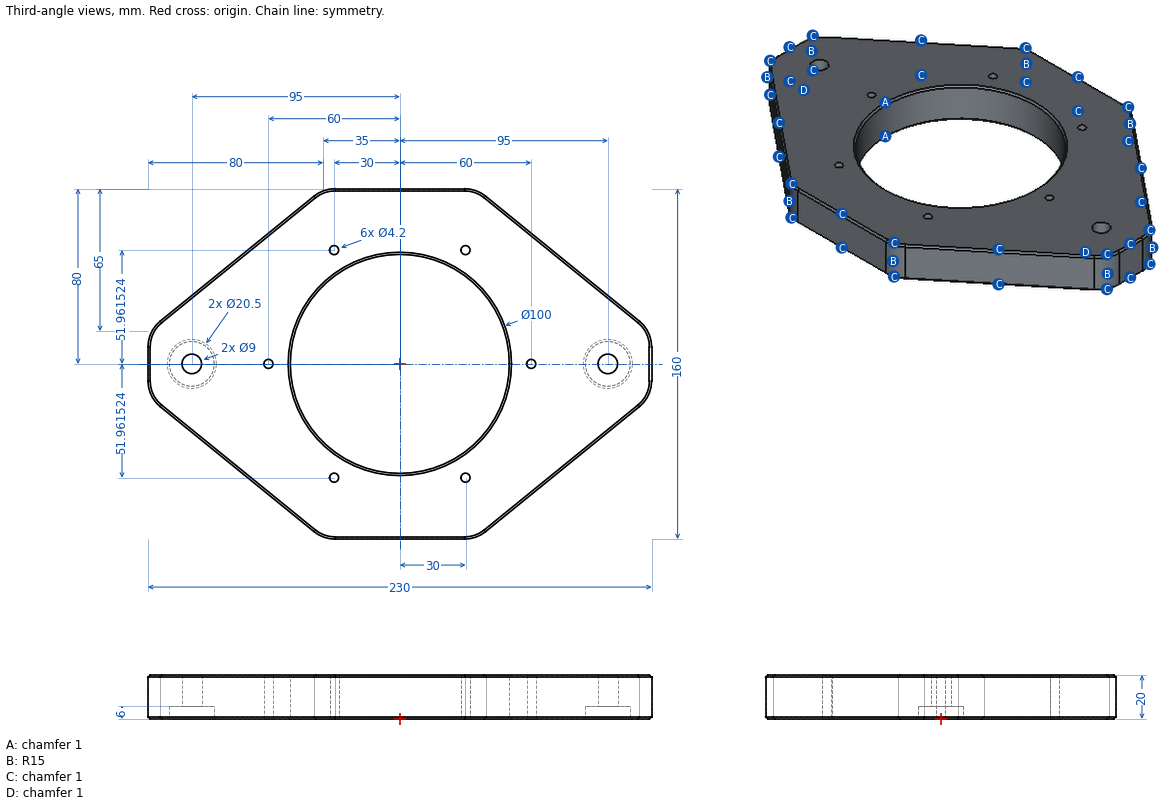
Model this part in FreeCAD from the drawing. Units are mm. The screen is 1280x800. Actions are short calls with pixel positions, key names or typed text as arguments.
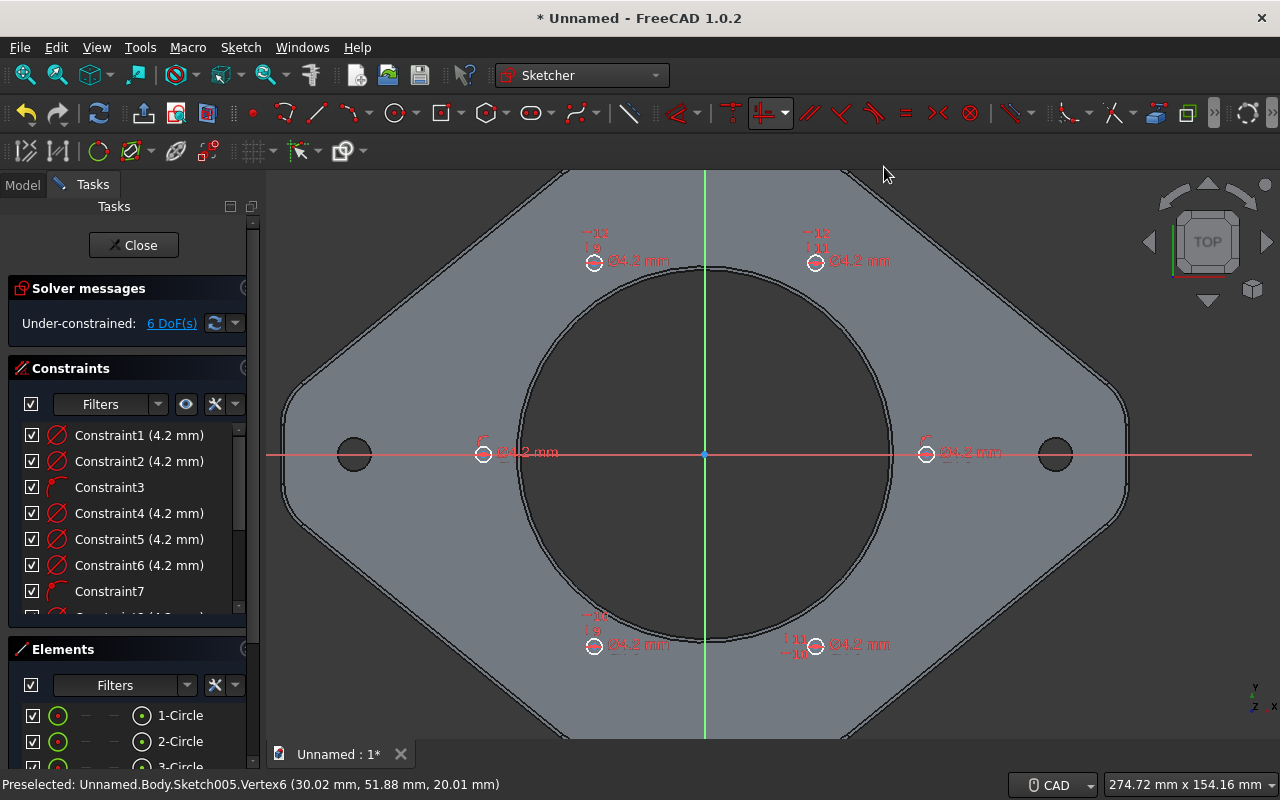
click(676, 114)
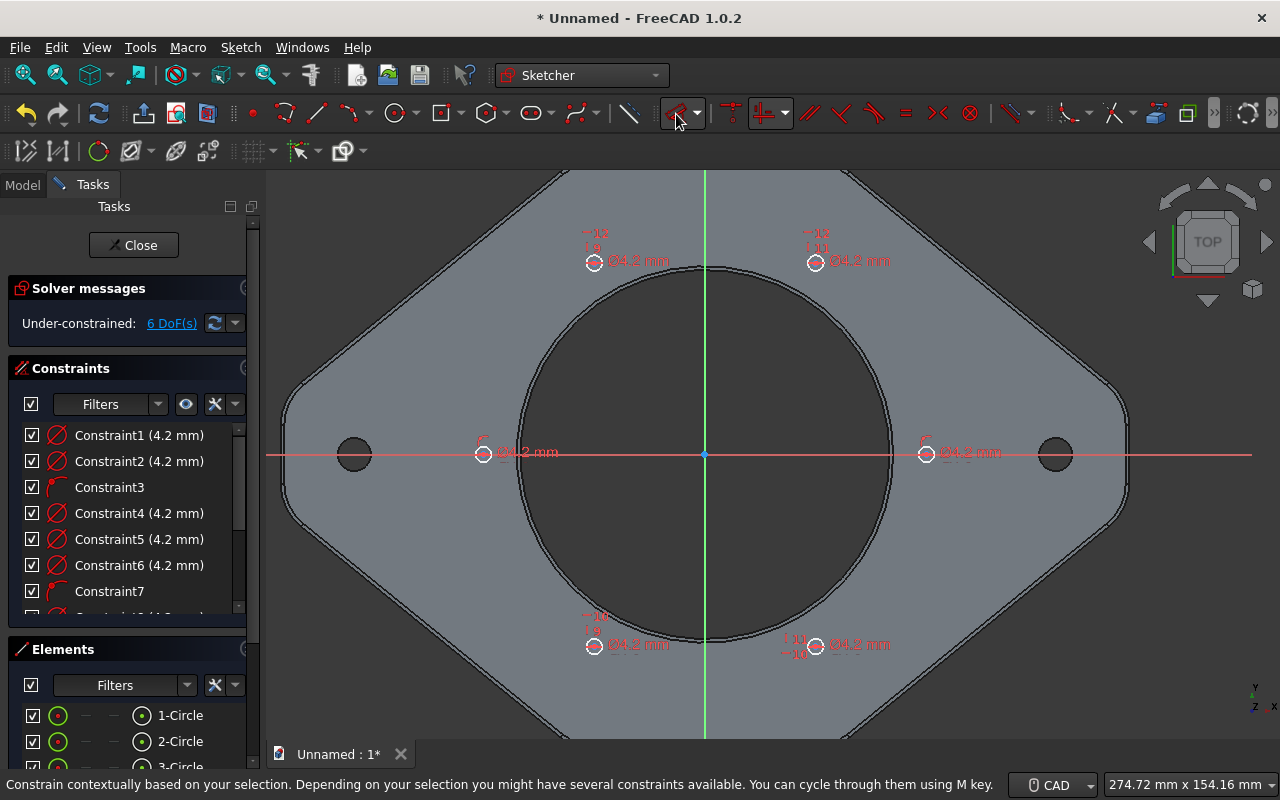
click(594, 263)
click(650, 229)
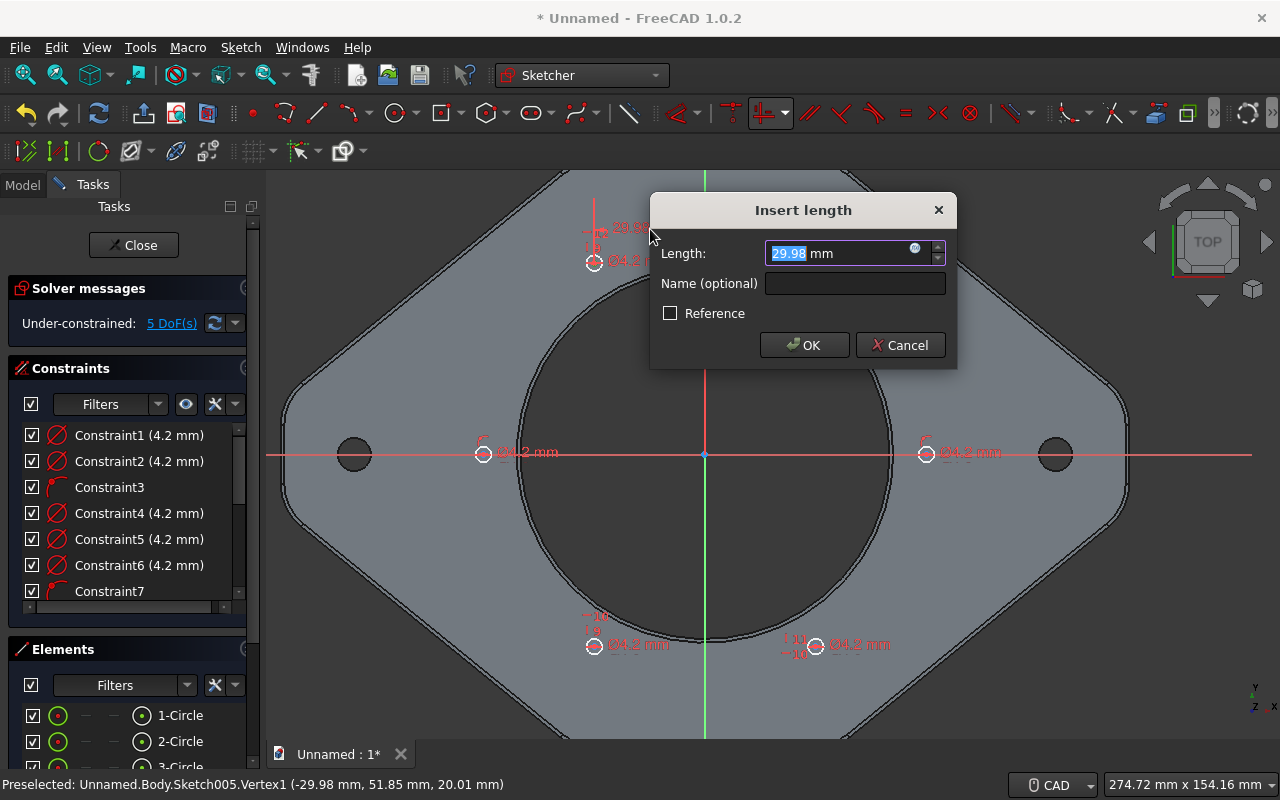
text(30)
key(Return)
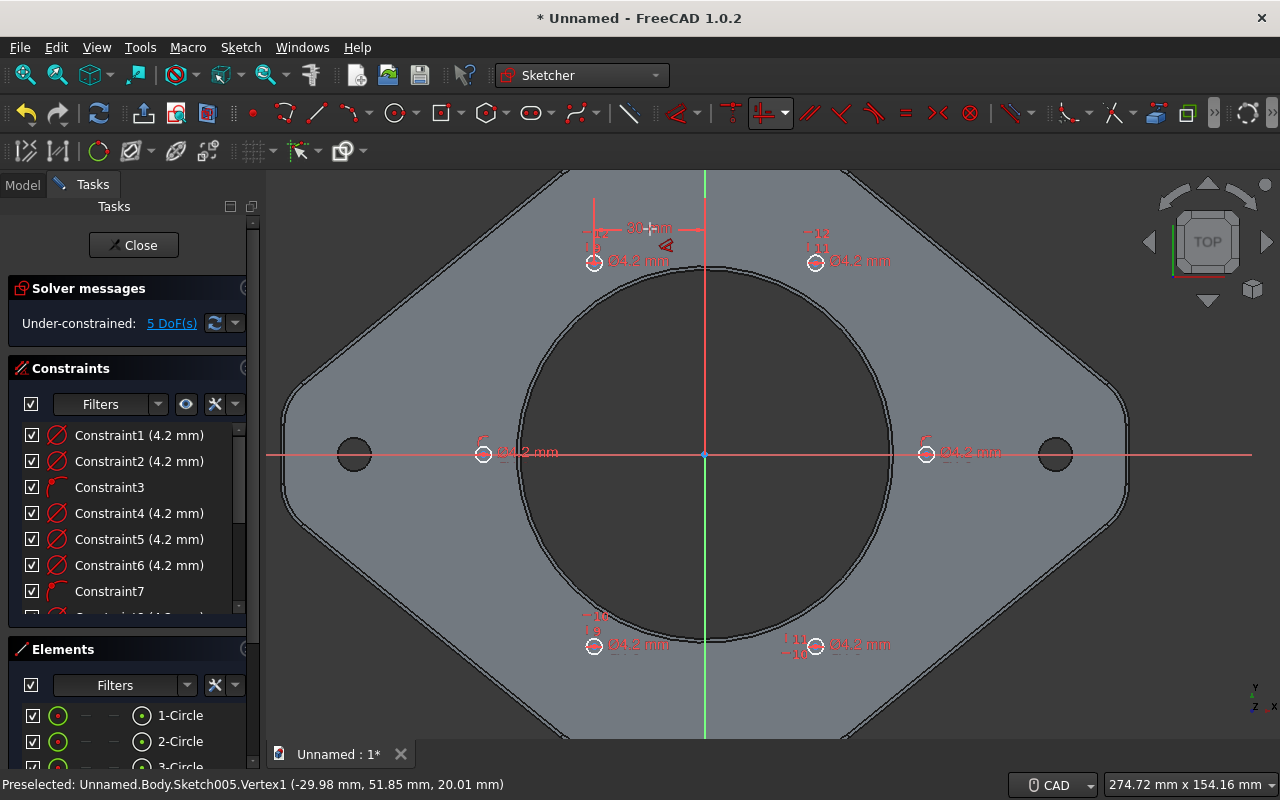
click(484, 454)
click(594, 488)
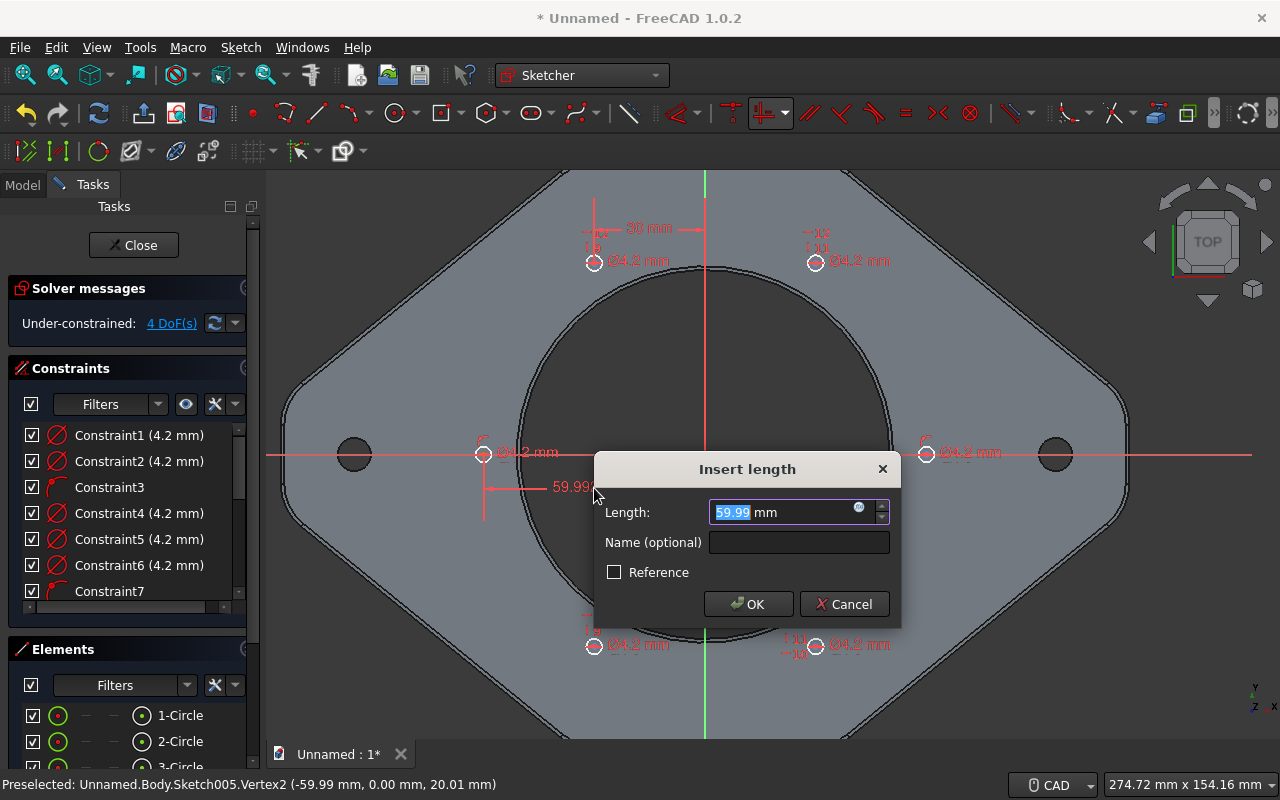
text(60)
key(Return)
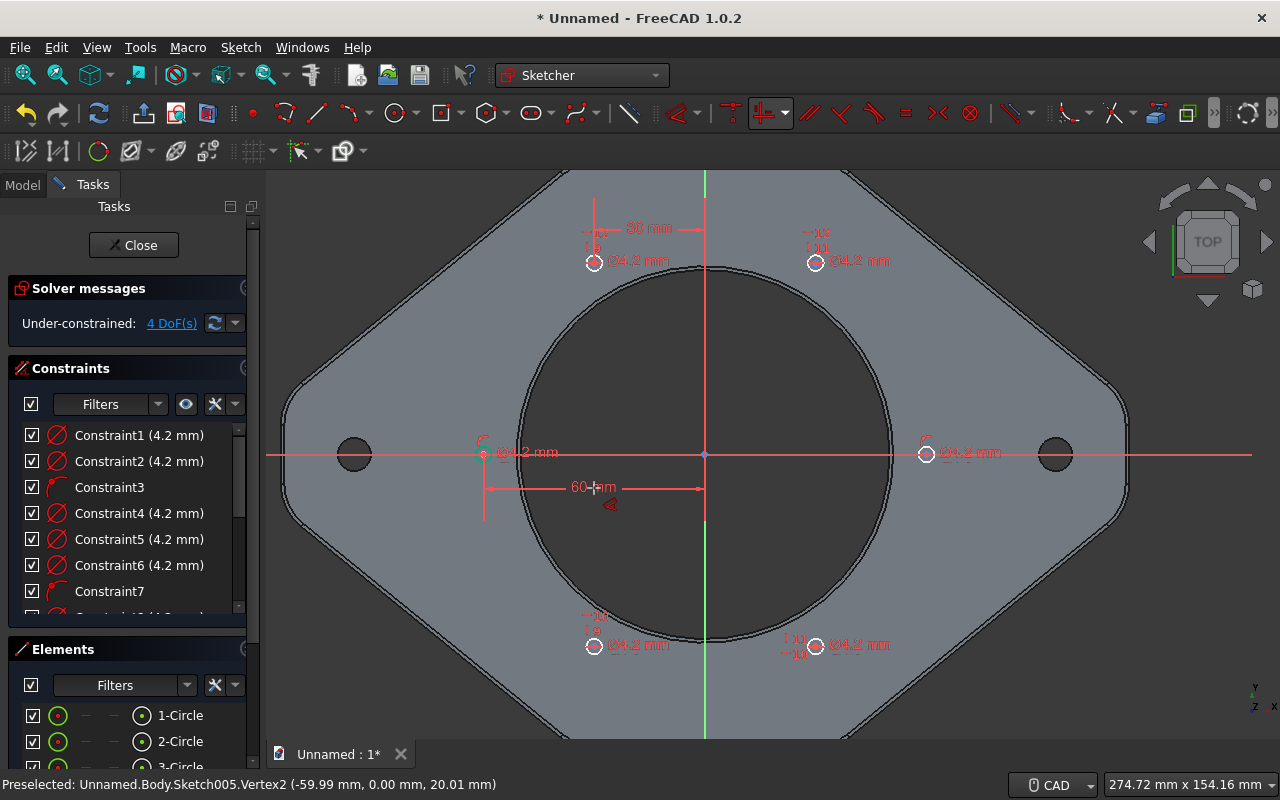
click(816, 647)
click(760, 681)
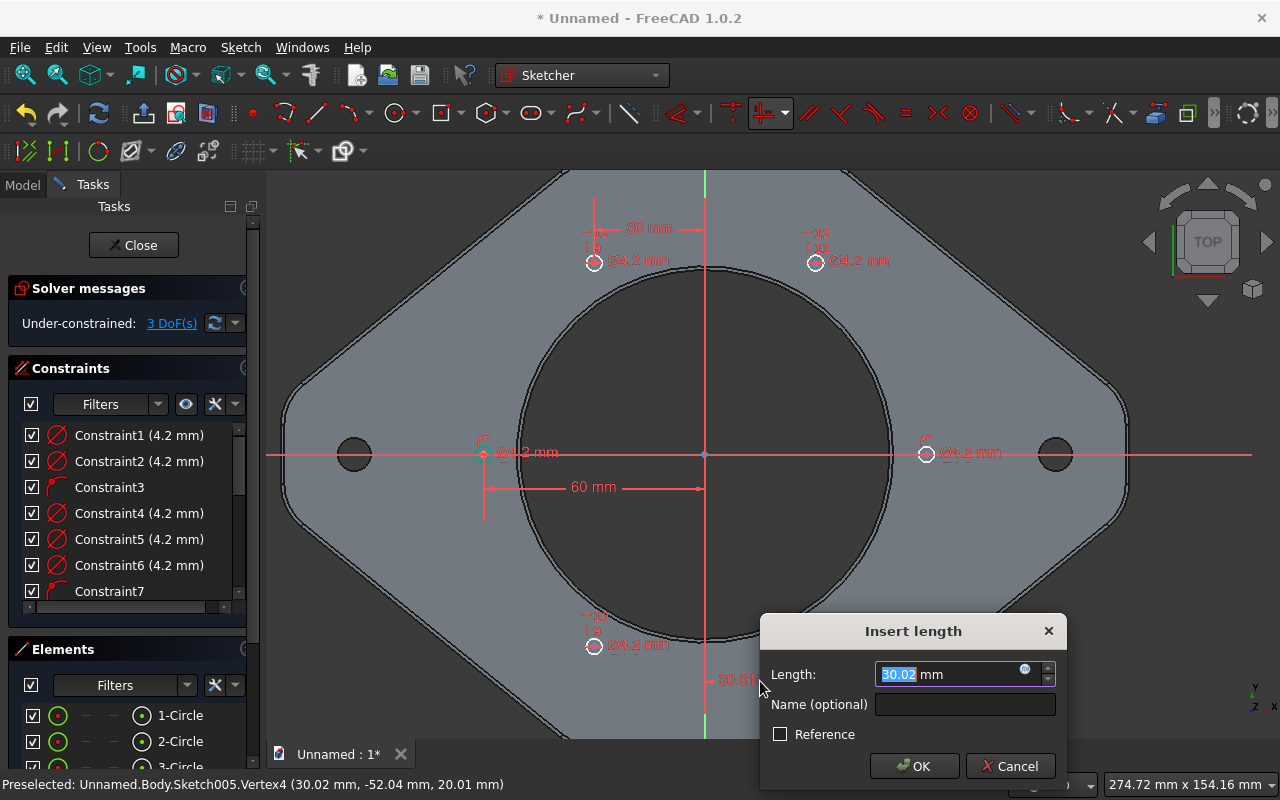
text(30)
key(Return)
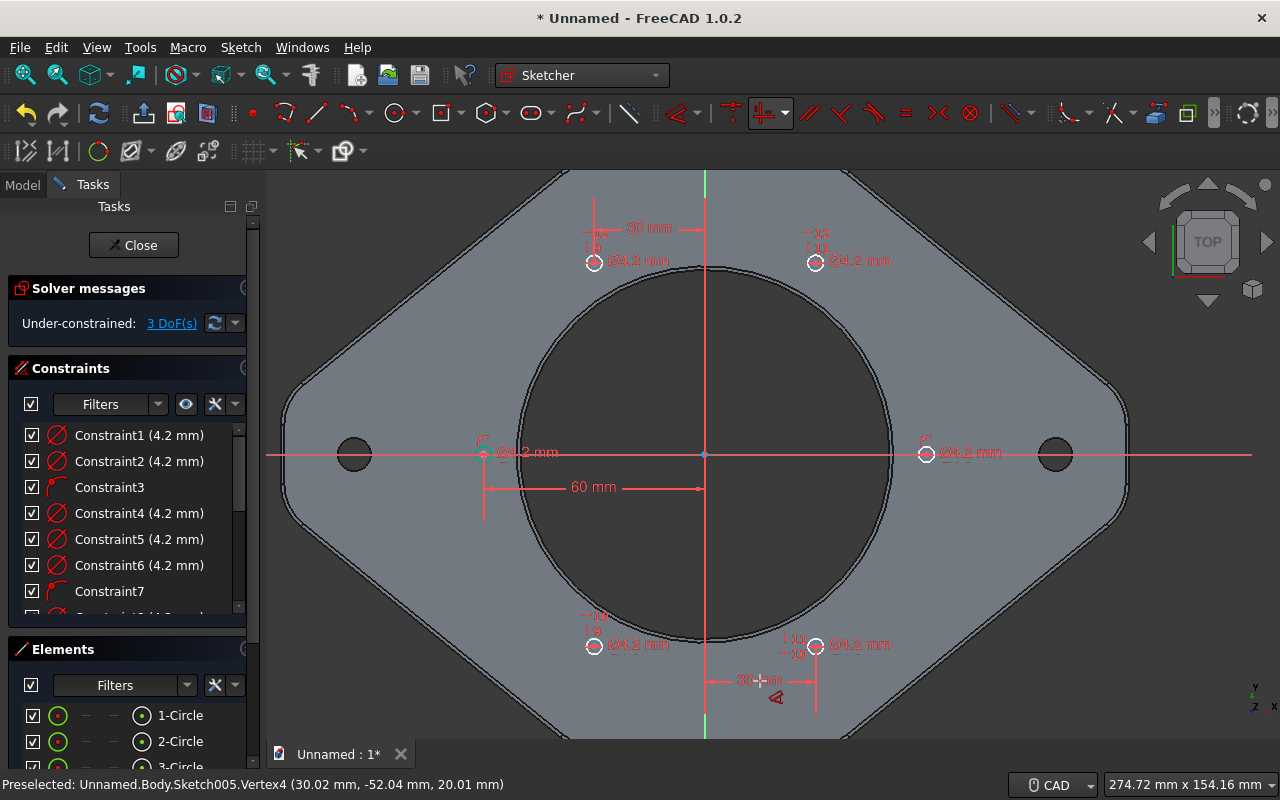
click(926, 454)
click(816, 488)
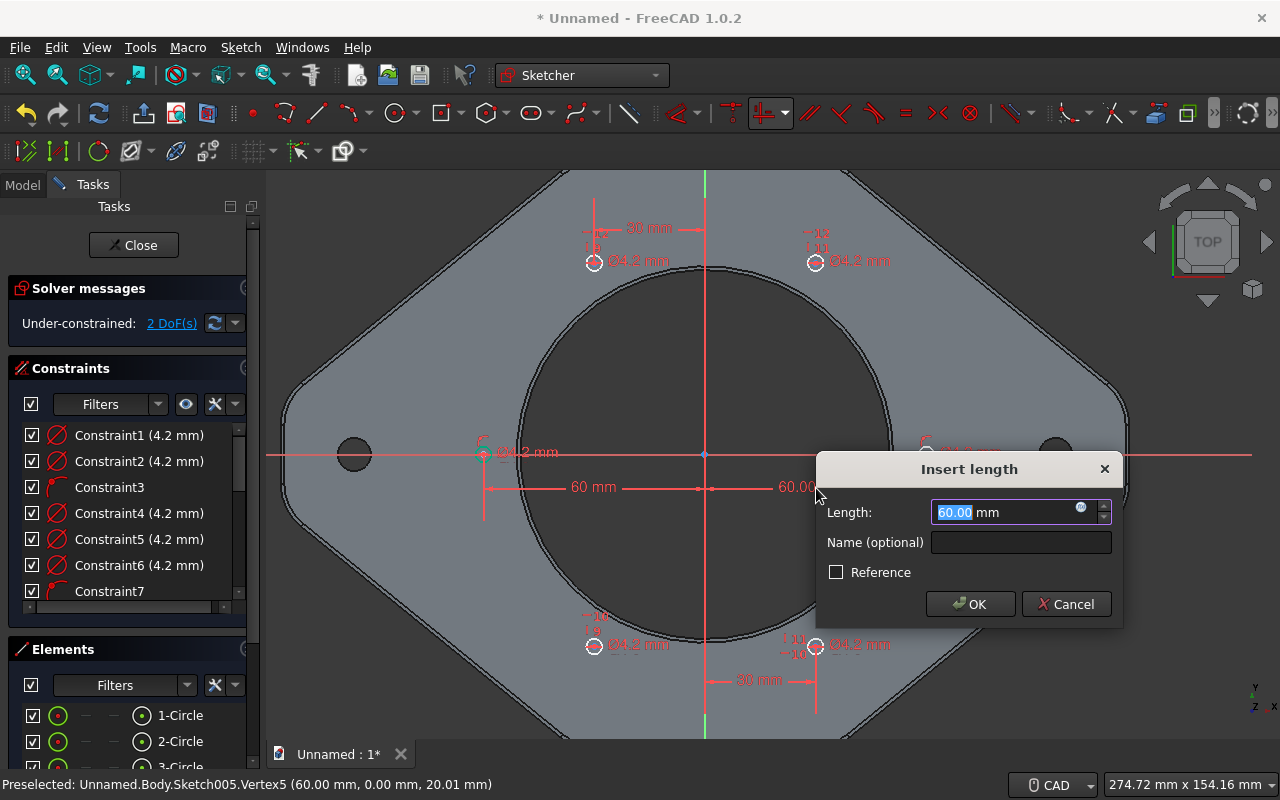
text(60)
key(Return)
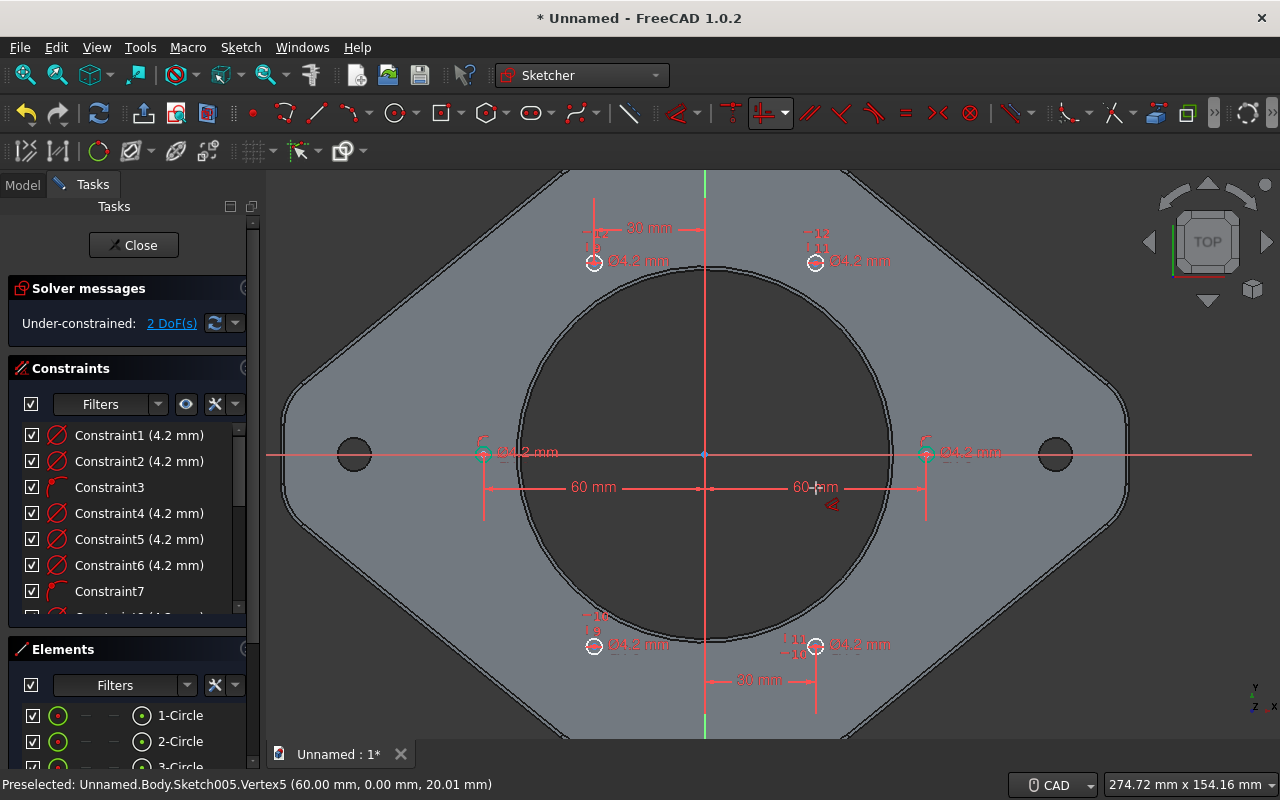
click(594, 263)
click(560, 359)